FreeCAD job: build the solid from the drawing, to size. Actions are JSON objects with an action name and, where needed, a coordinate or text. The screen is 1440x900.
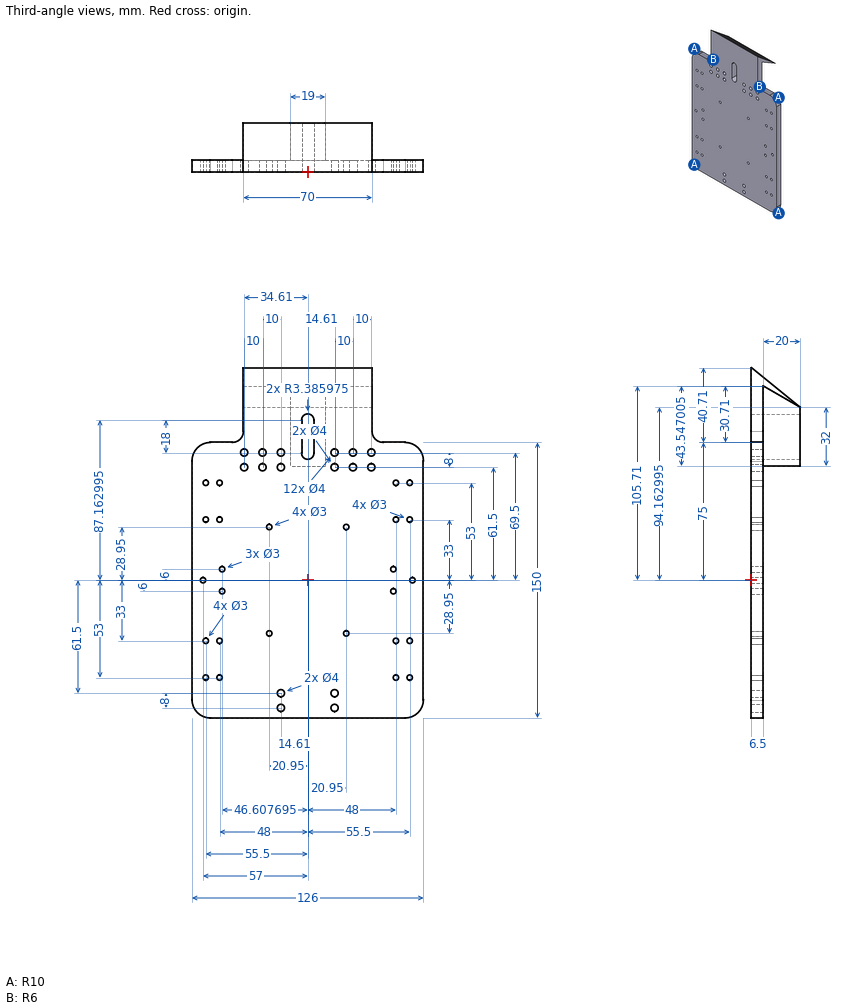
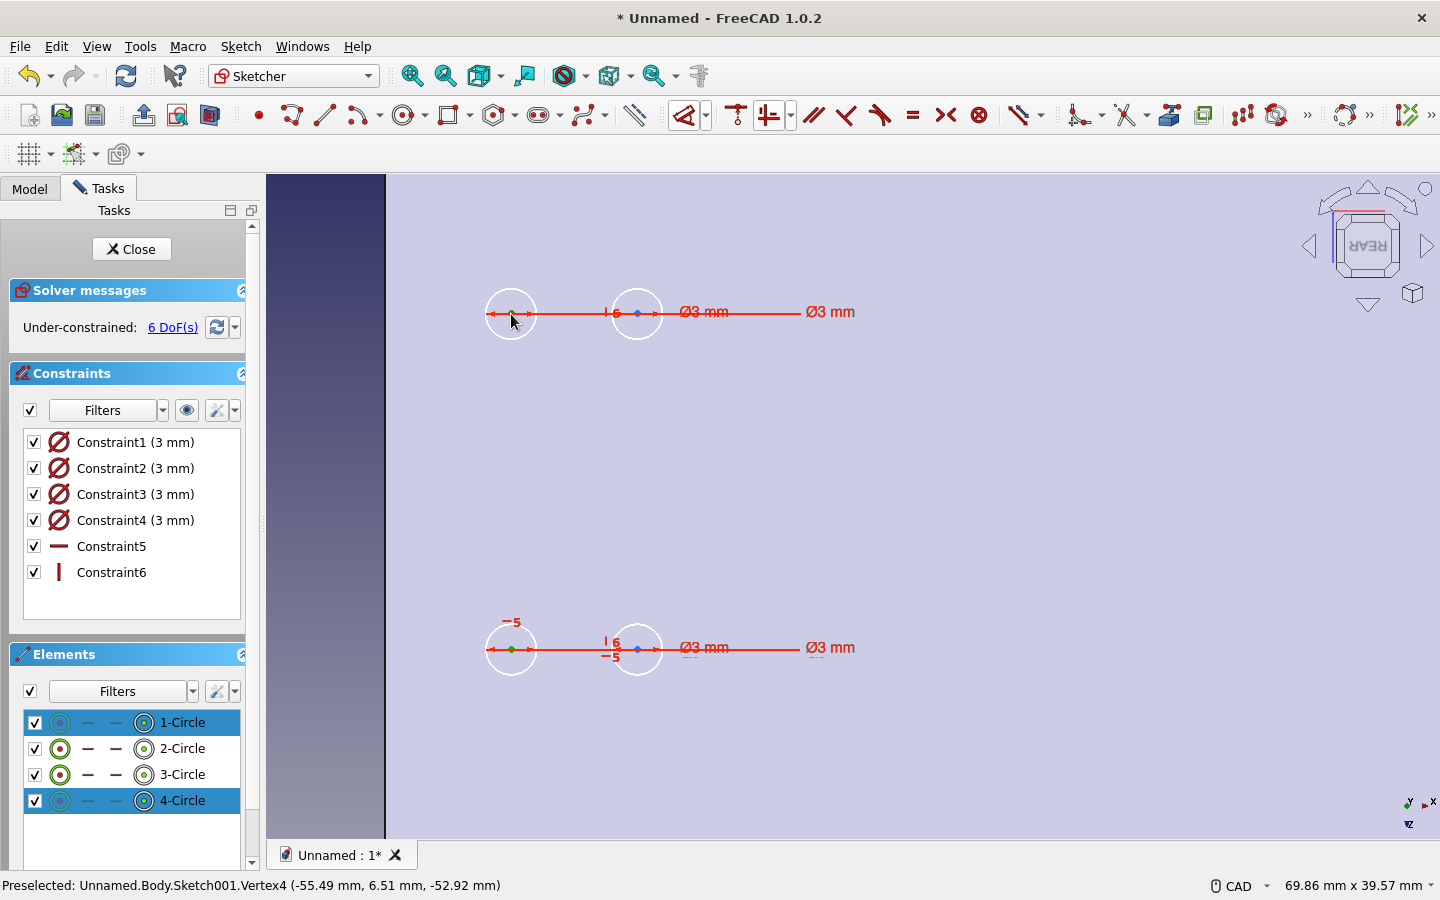
{"action": "key", "text": "v"}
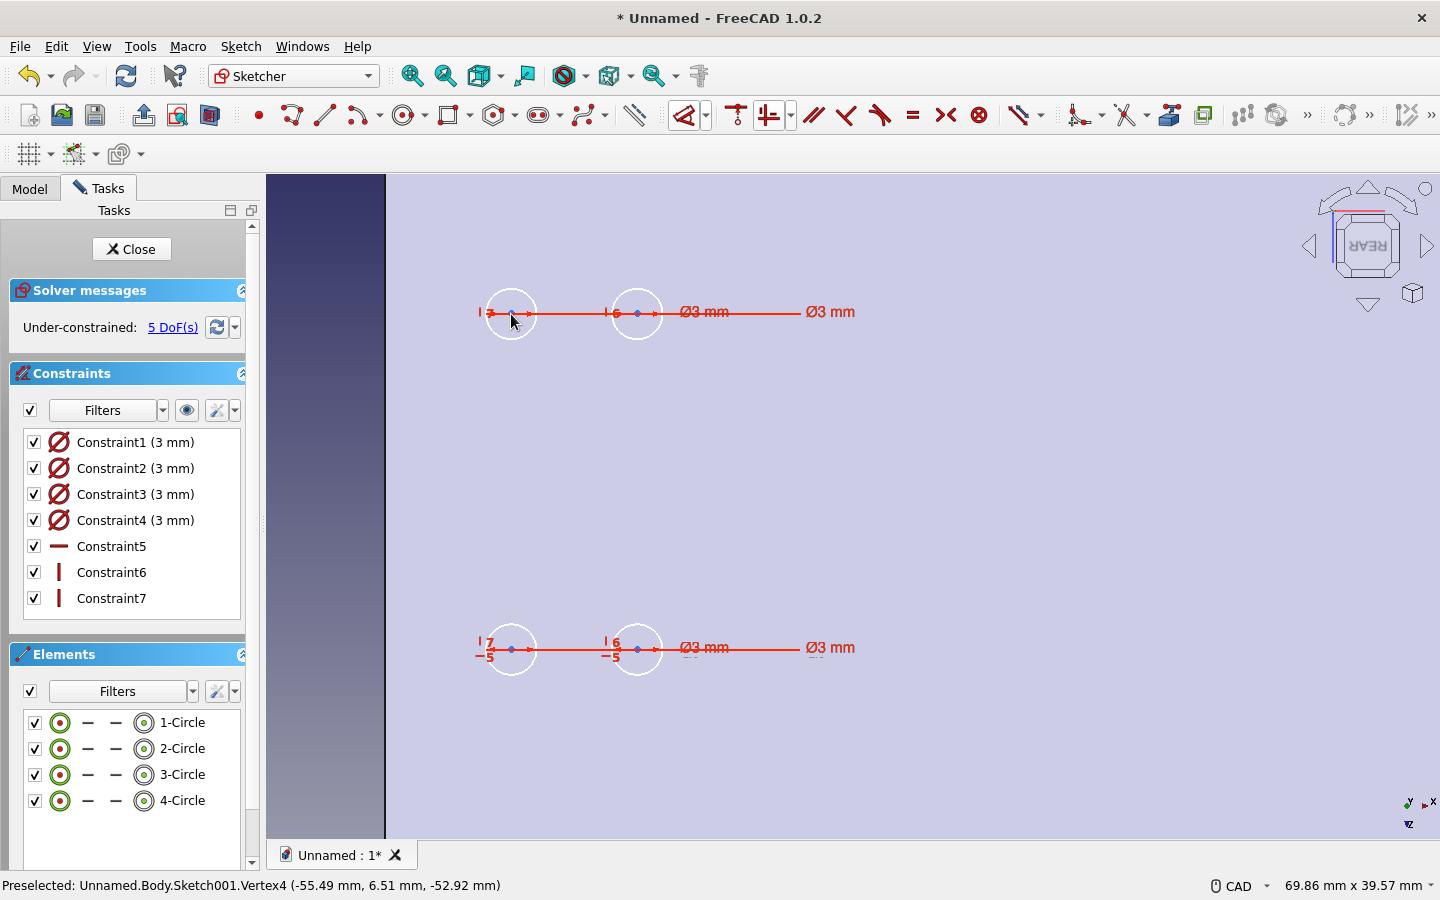
{"action": "left_click", "coordinate": [637, 314]}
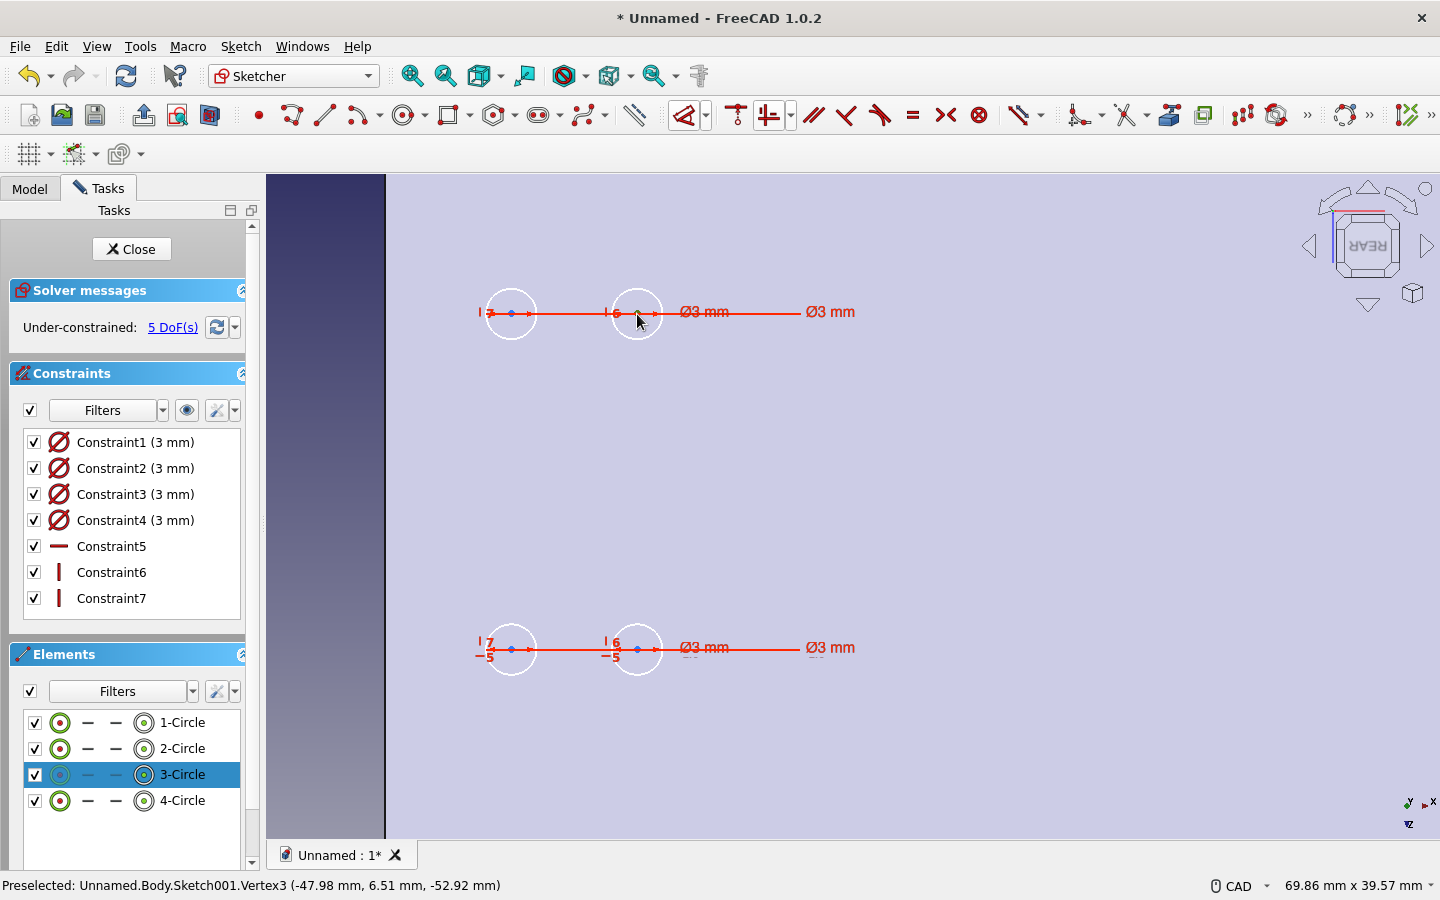
{"action": "left_click", "coordinate": [511, 314]}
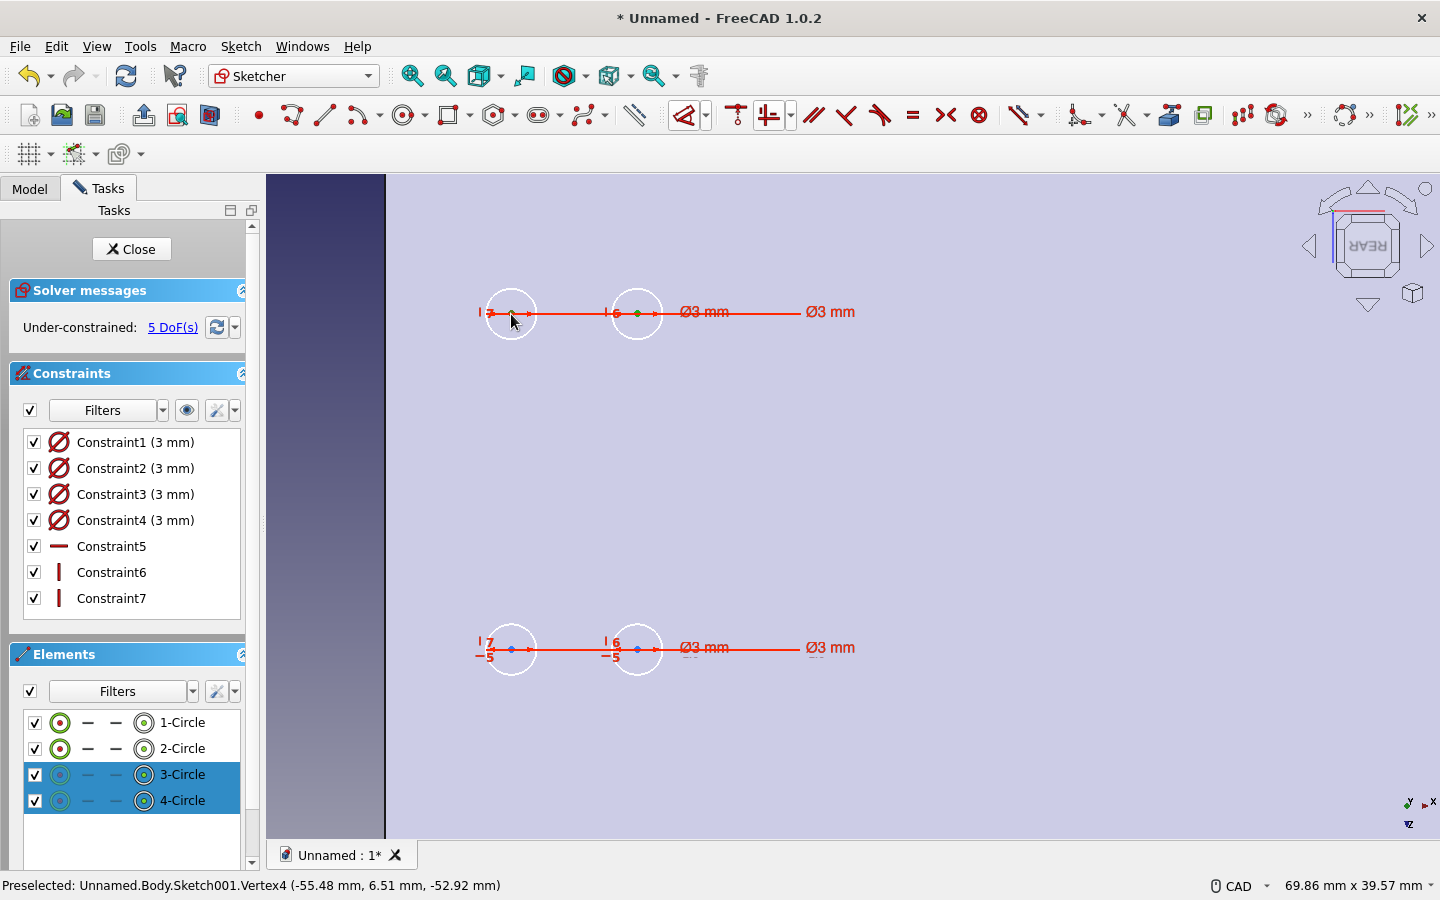
{"action": "left_click", "coordinate": [790, 116]}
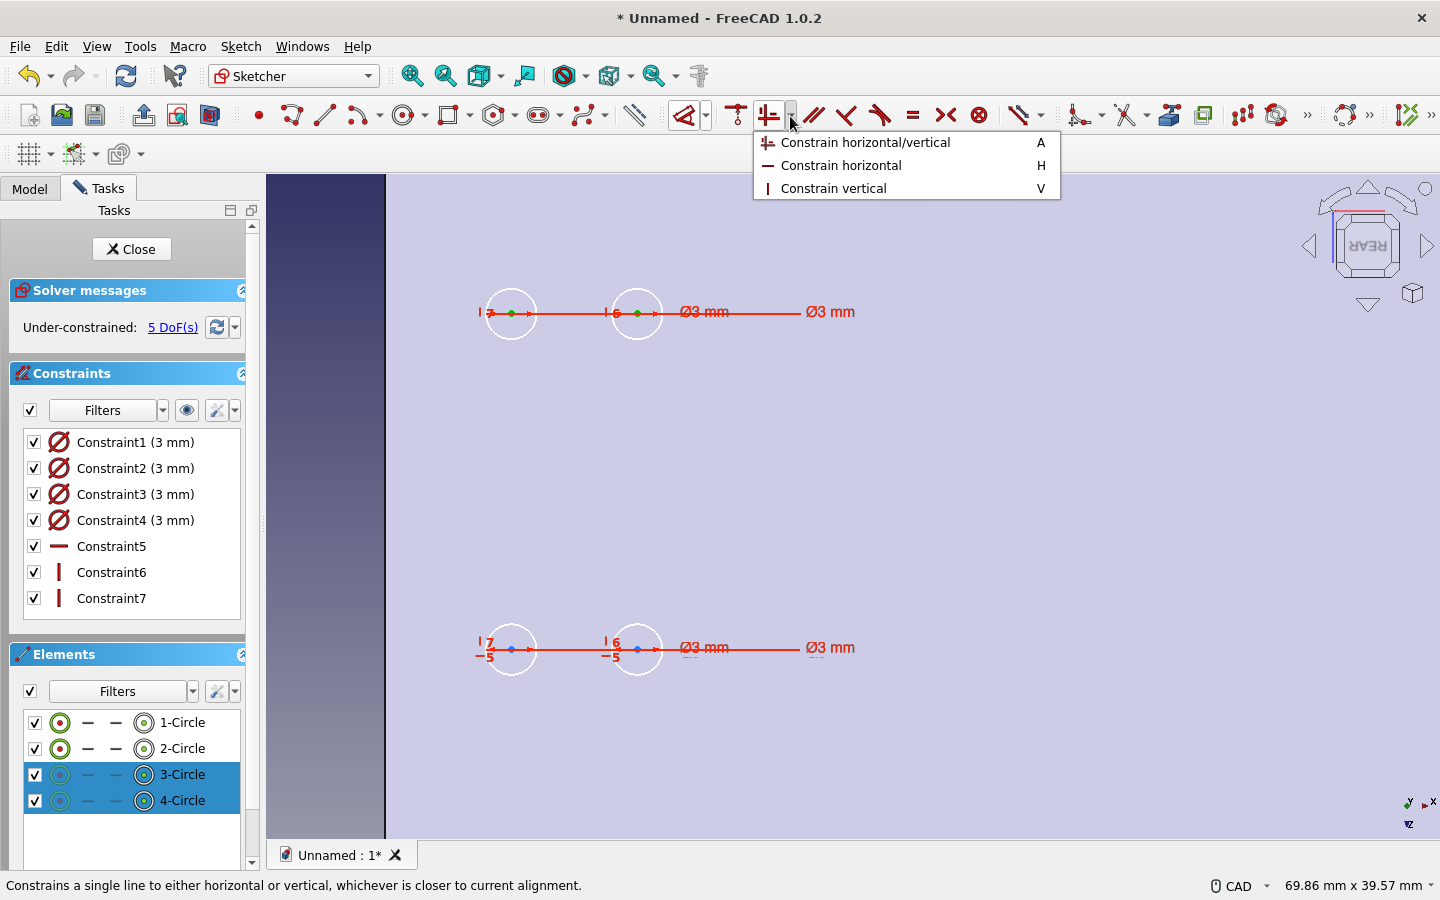
{"action": "left_click", "coordinate": [907, 166]}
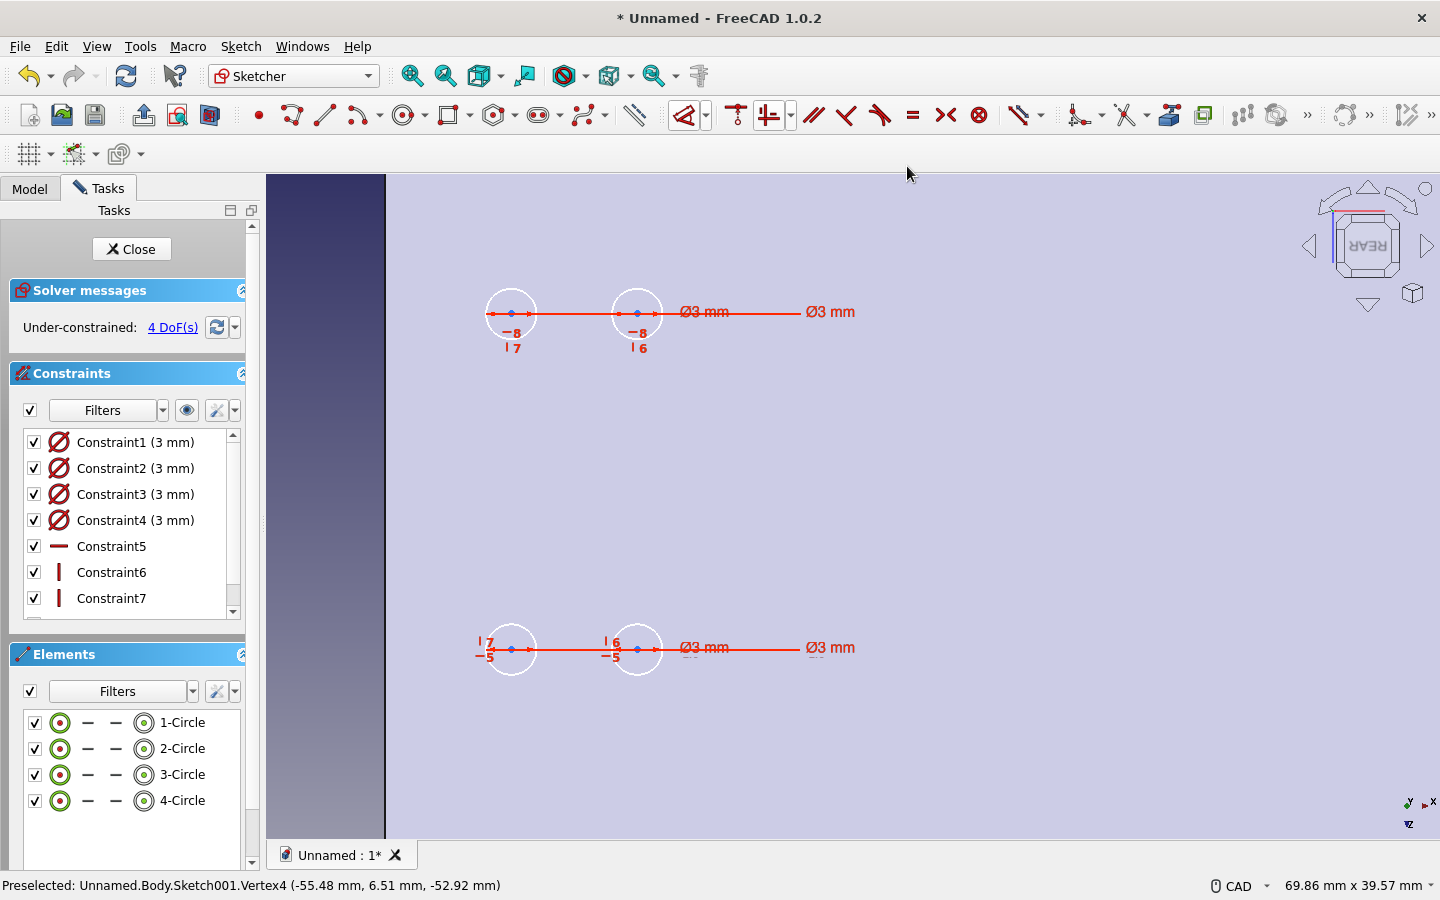
{"action": "left_click", "coordinate": [684, 116]}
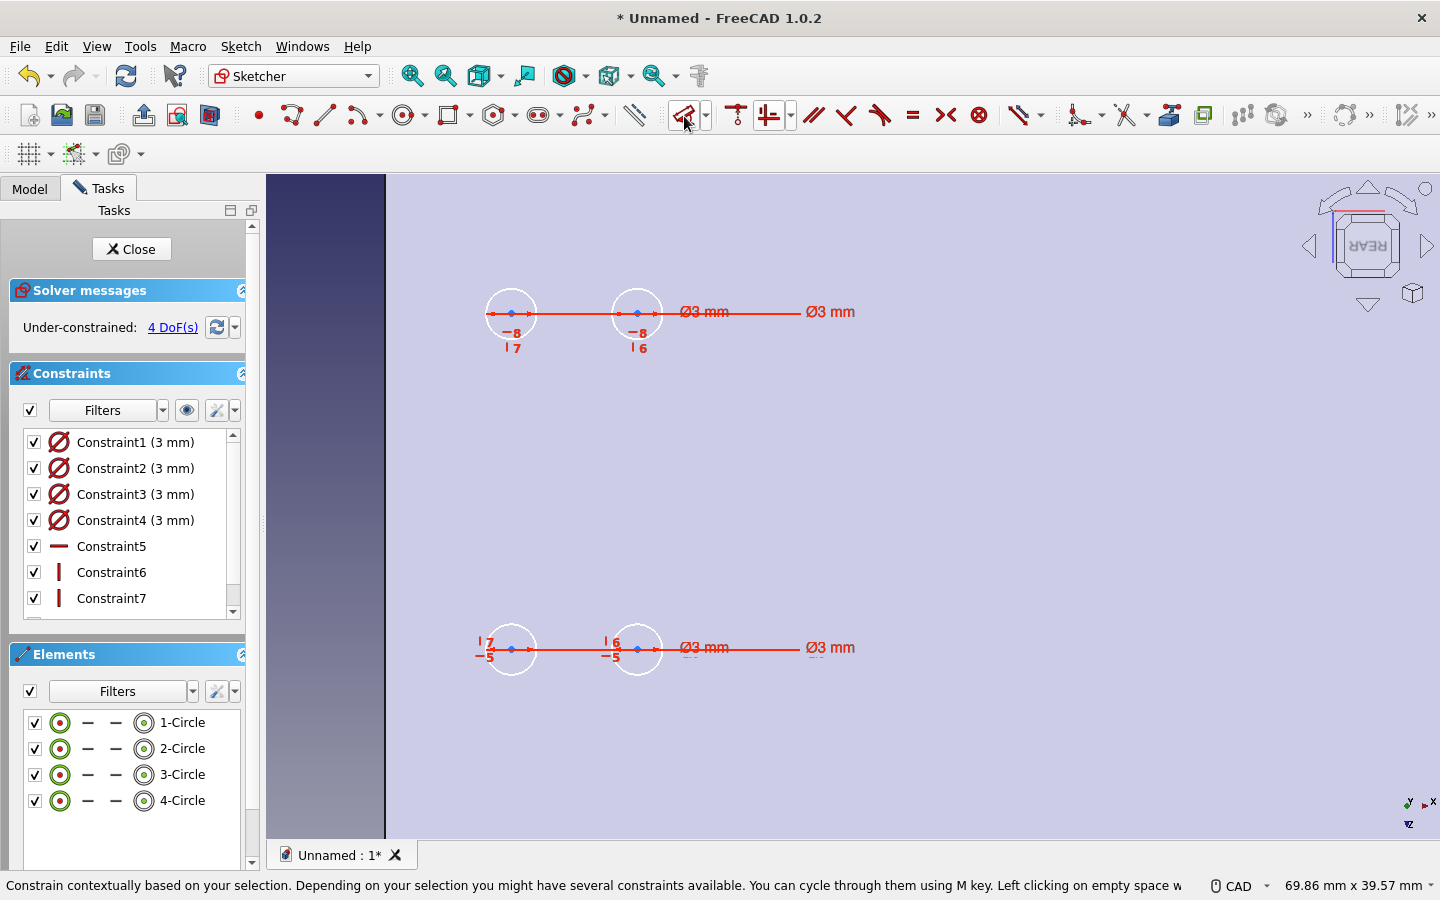
{"action": "left_click", "coordinate": [511, 650]}
{"action": "left_click", "coordinate": [477, 730]}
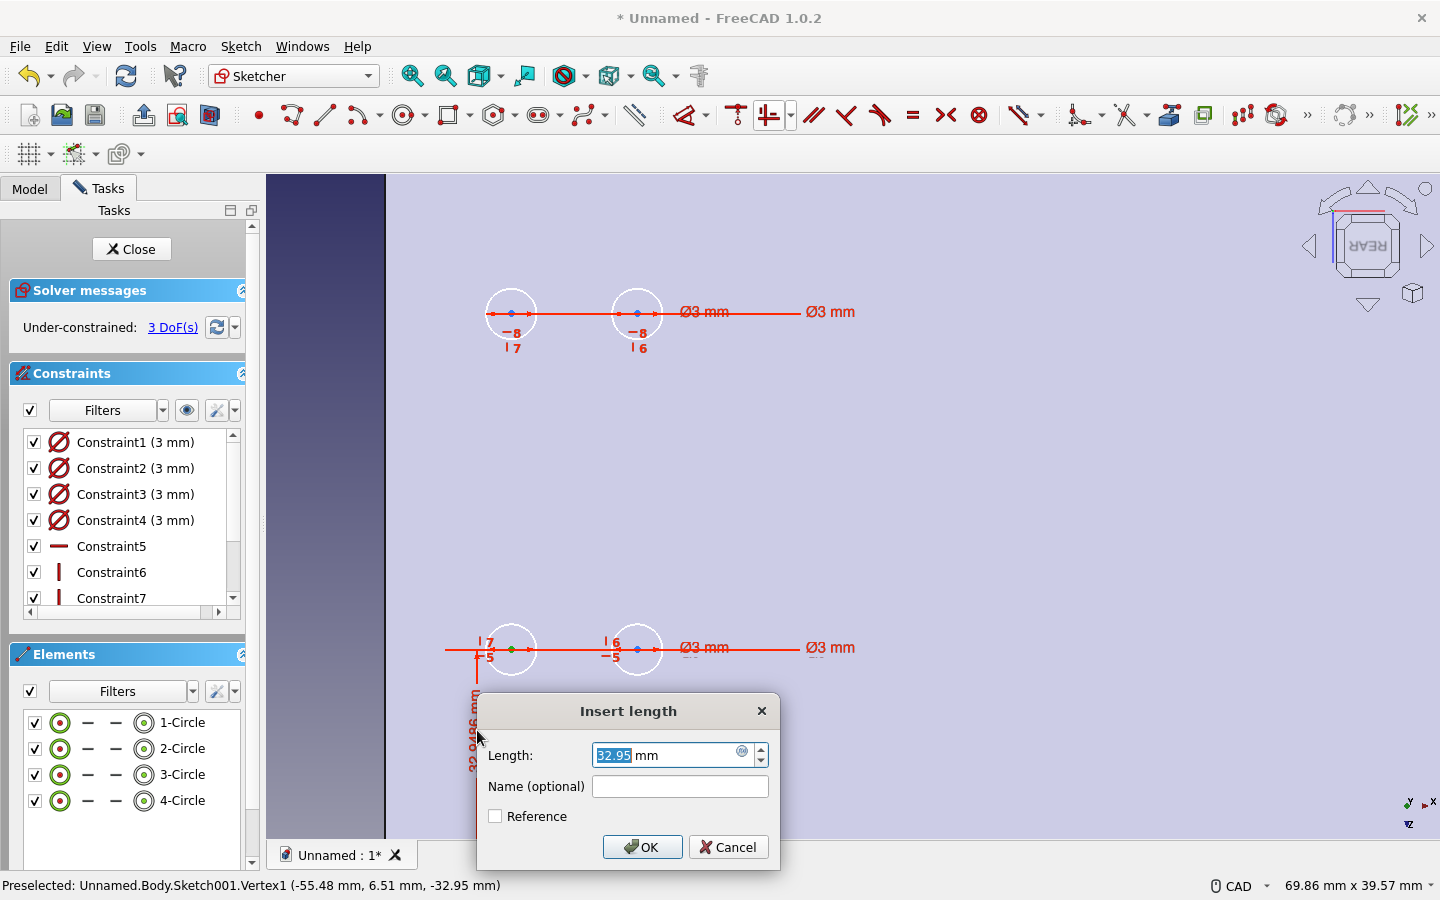
{"action": "type", "text": "33"}
{"action": "key", "text": "Return"}